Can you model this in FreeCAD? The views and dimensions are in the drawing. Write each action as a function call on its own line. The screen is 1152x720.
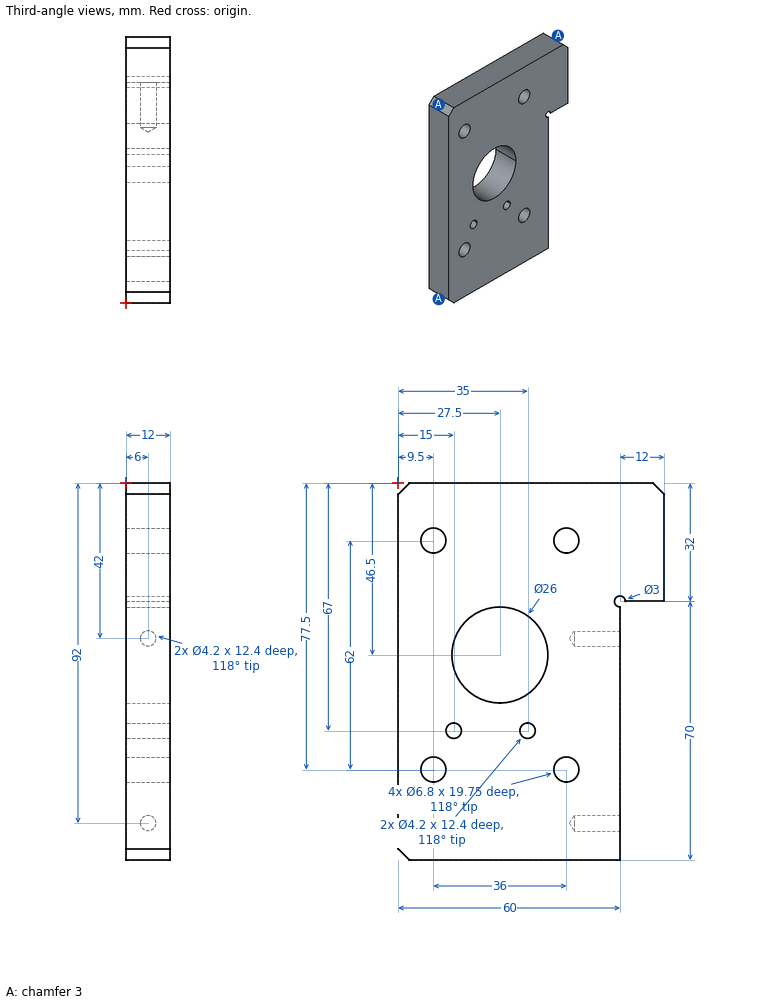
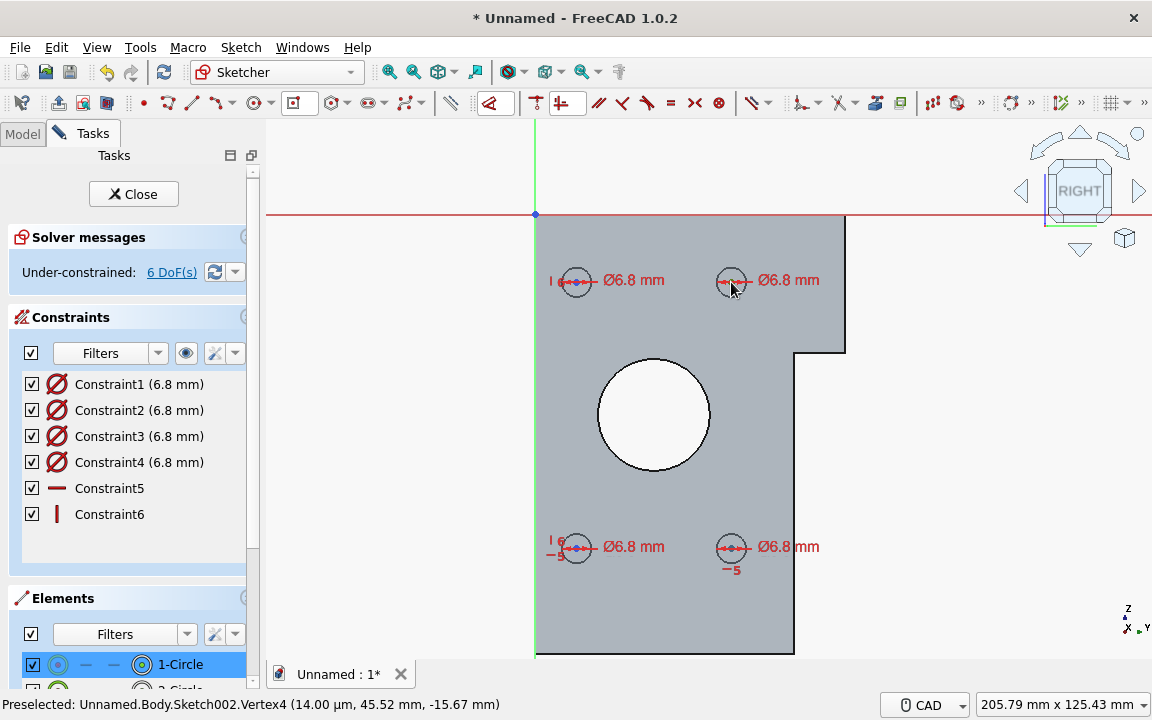
click(580, 104)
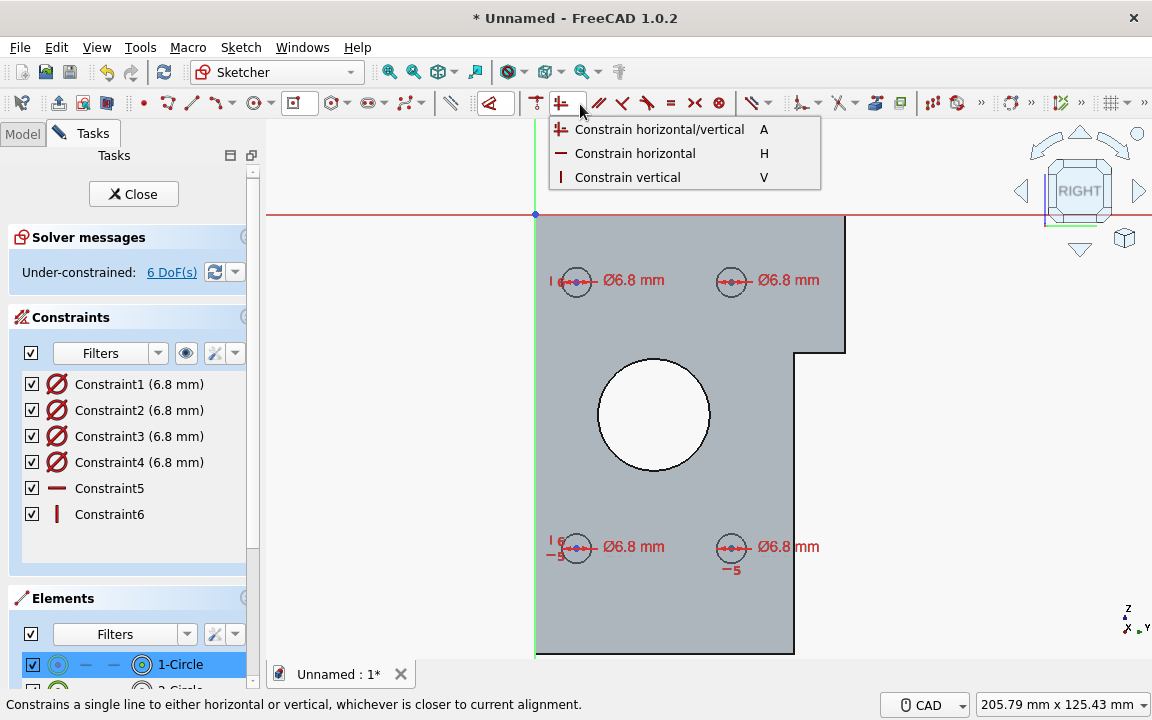
click(685, 177)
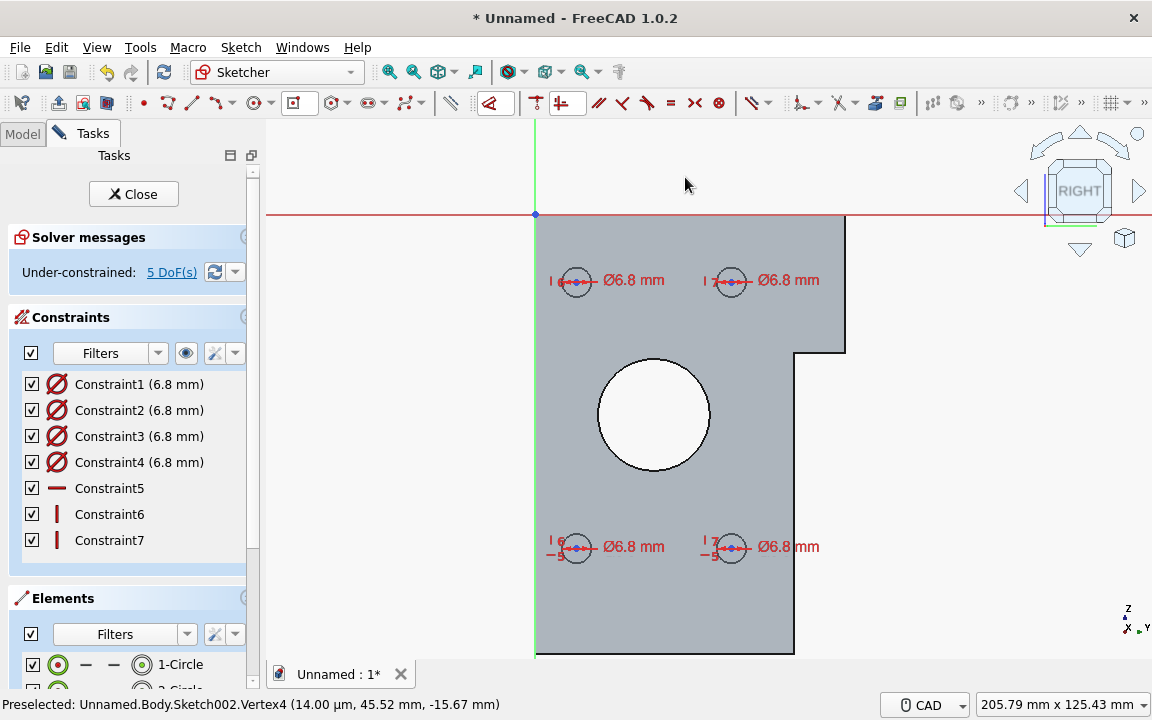
click(577, 282)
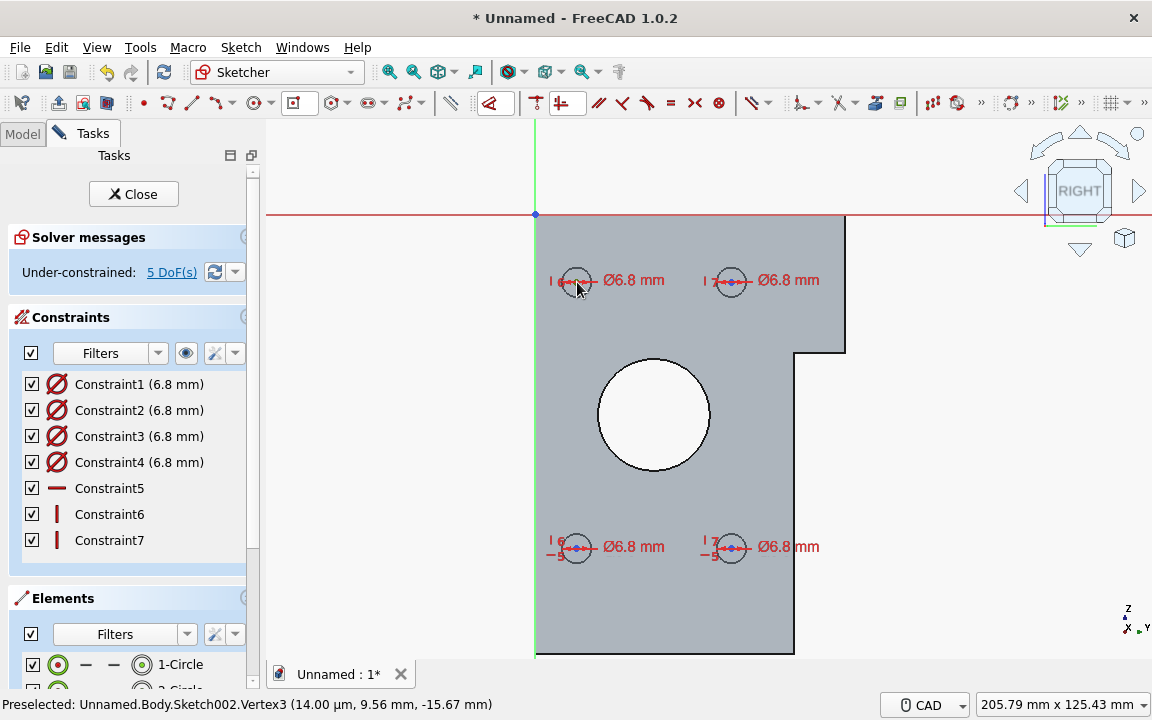
click(731, 282)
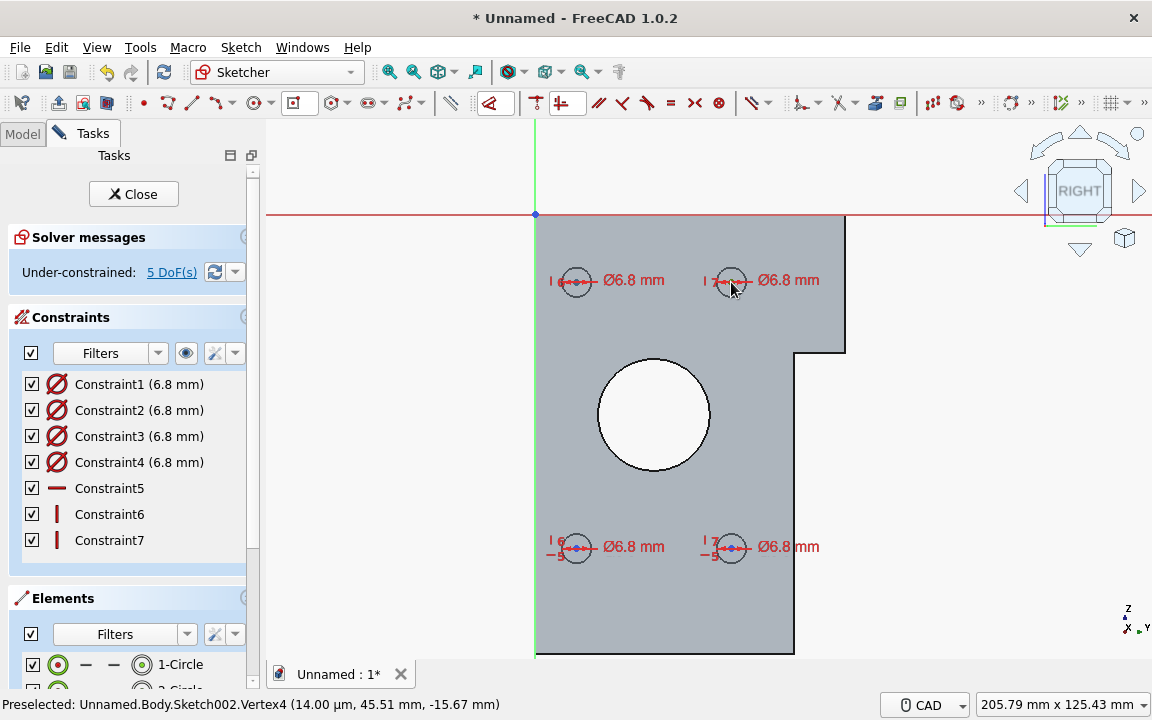
click(580, 104)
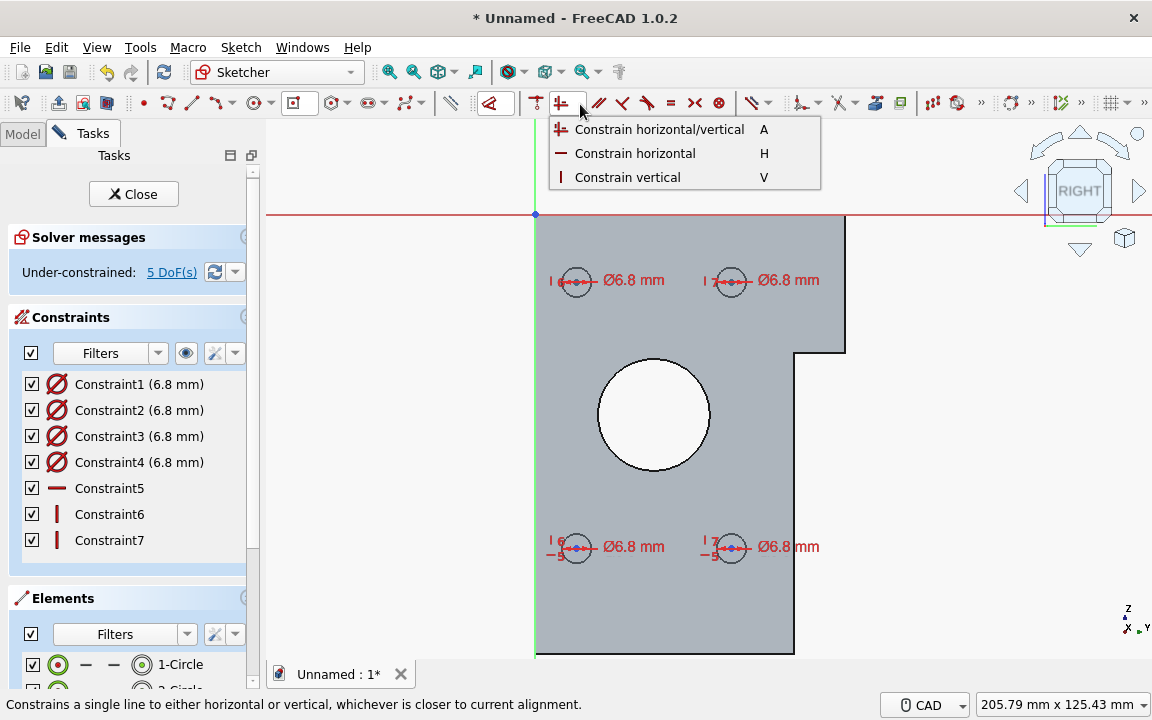
click(685, 153)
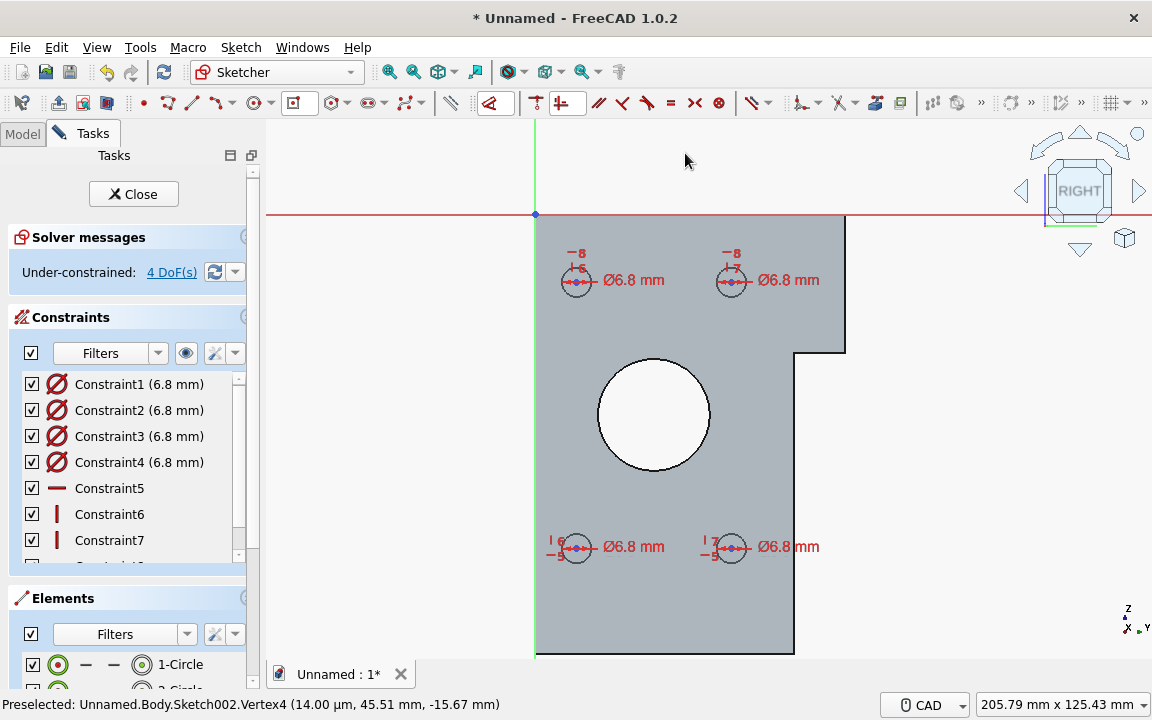
click(577, 549)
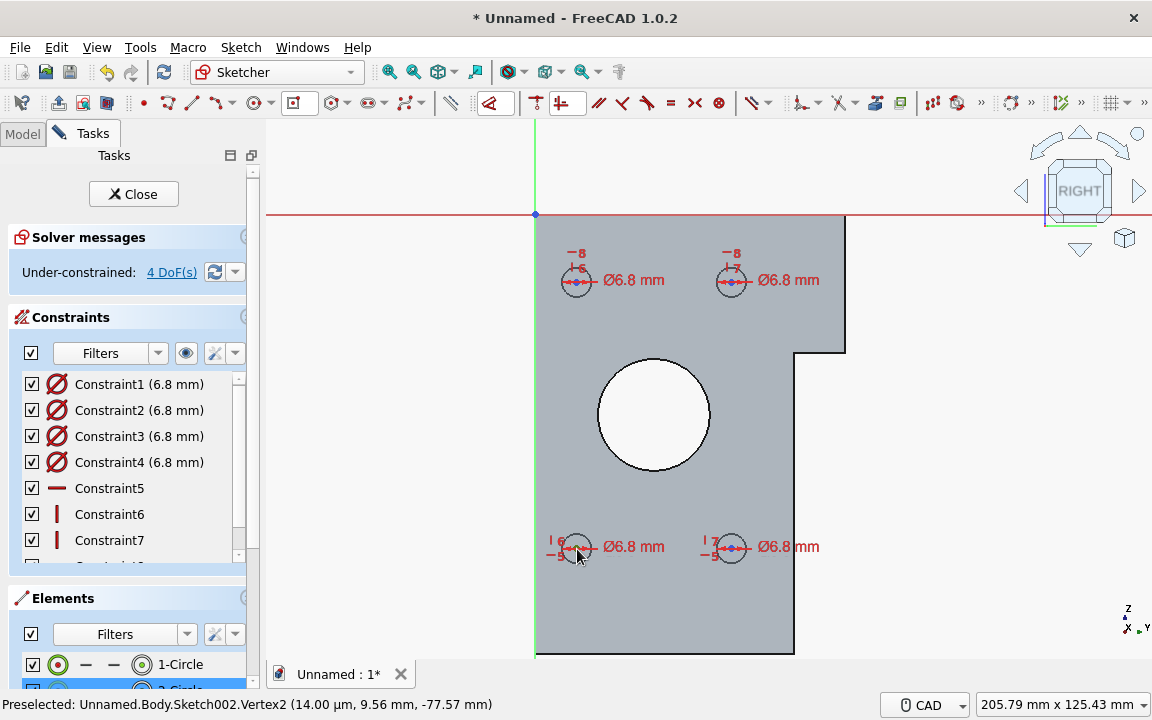
key(l)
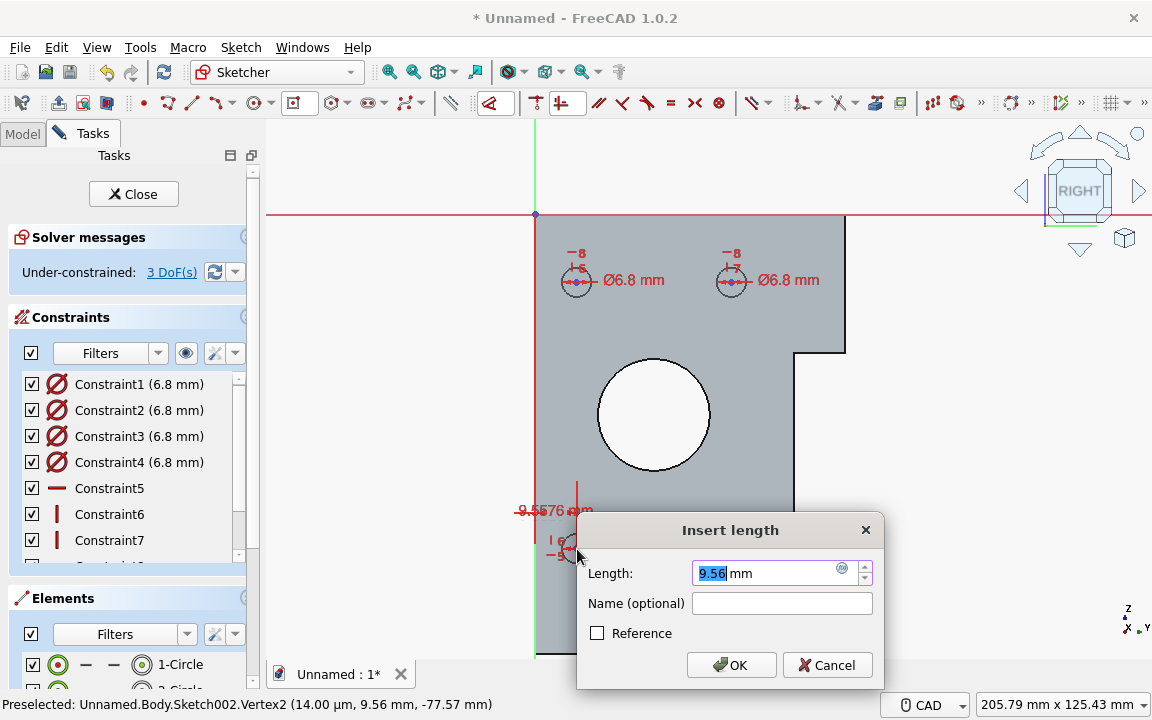
text(9.5)
key(Return)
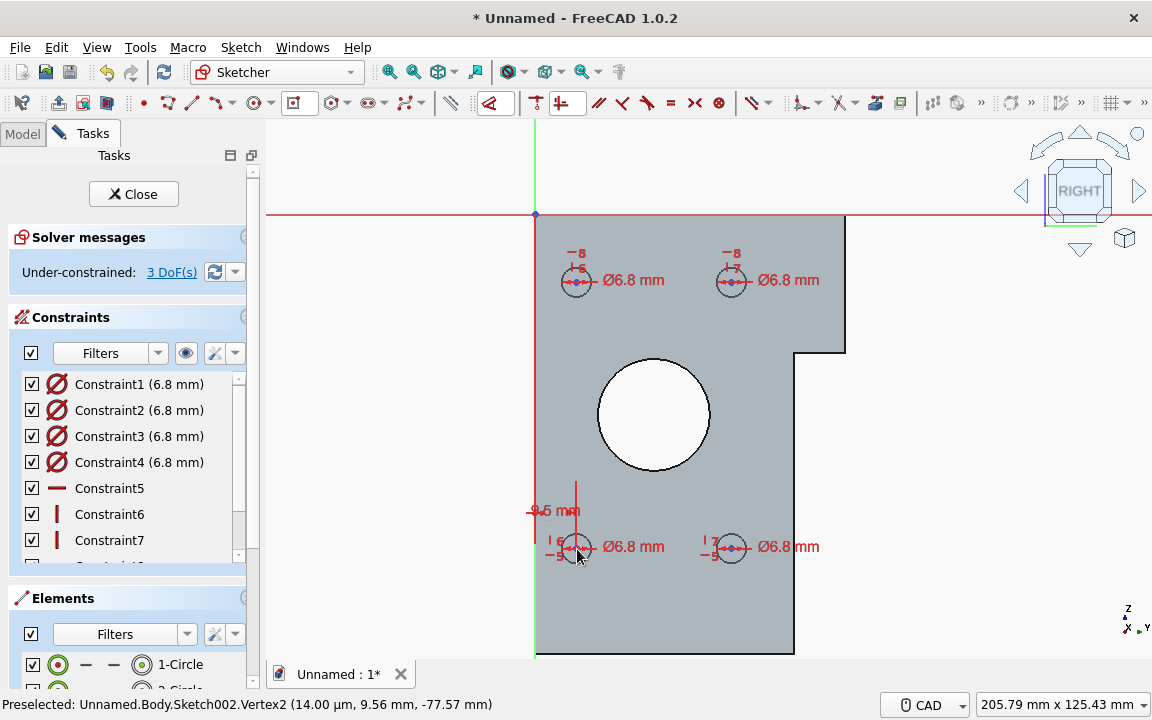
click(731, 549)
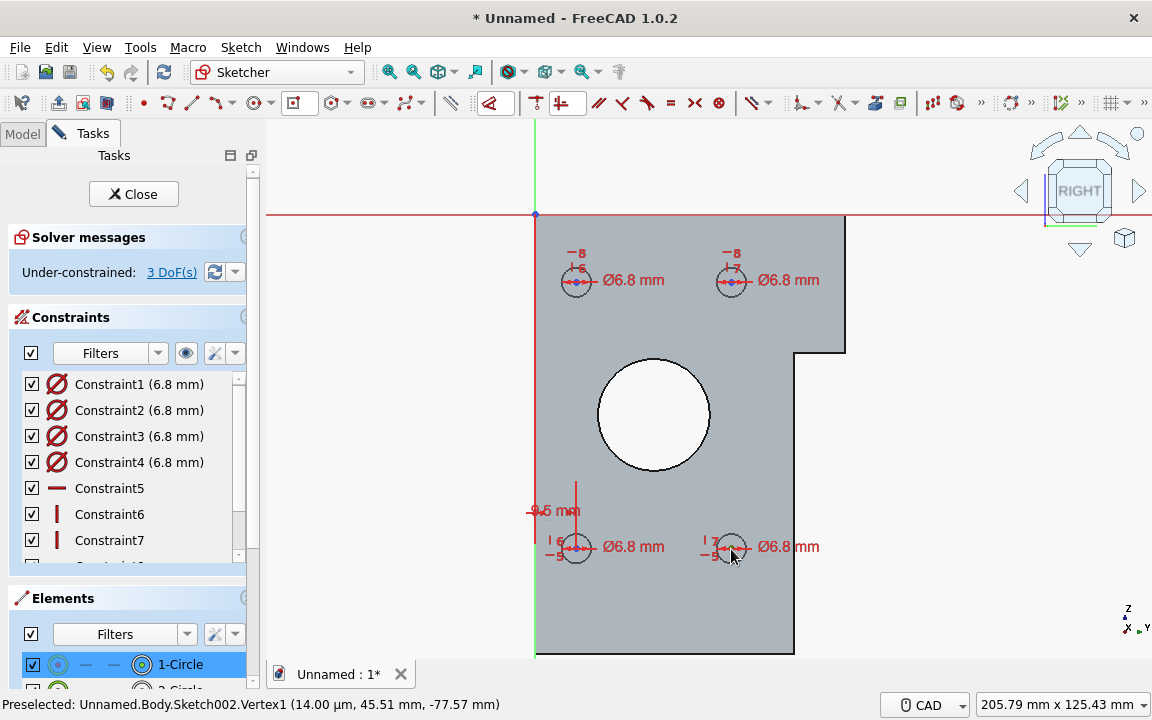
click(576, 549)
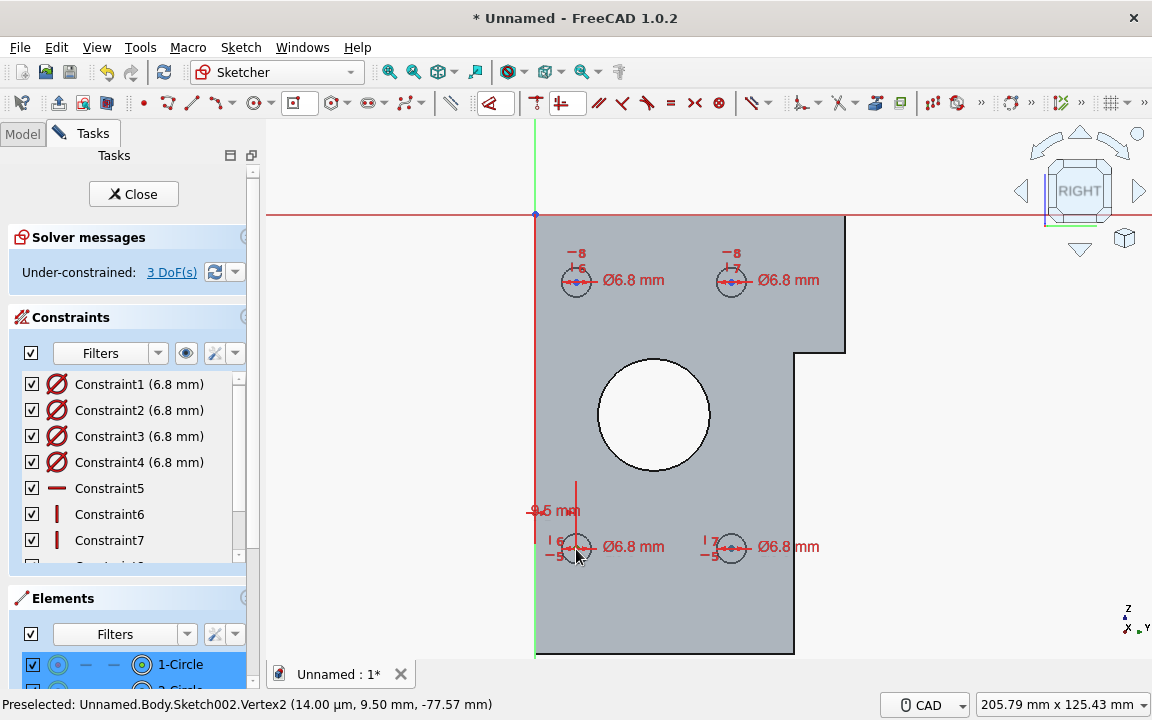
click(508, 104)